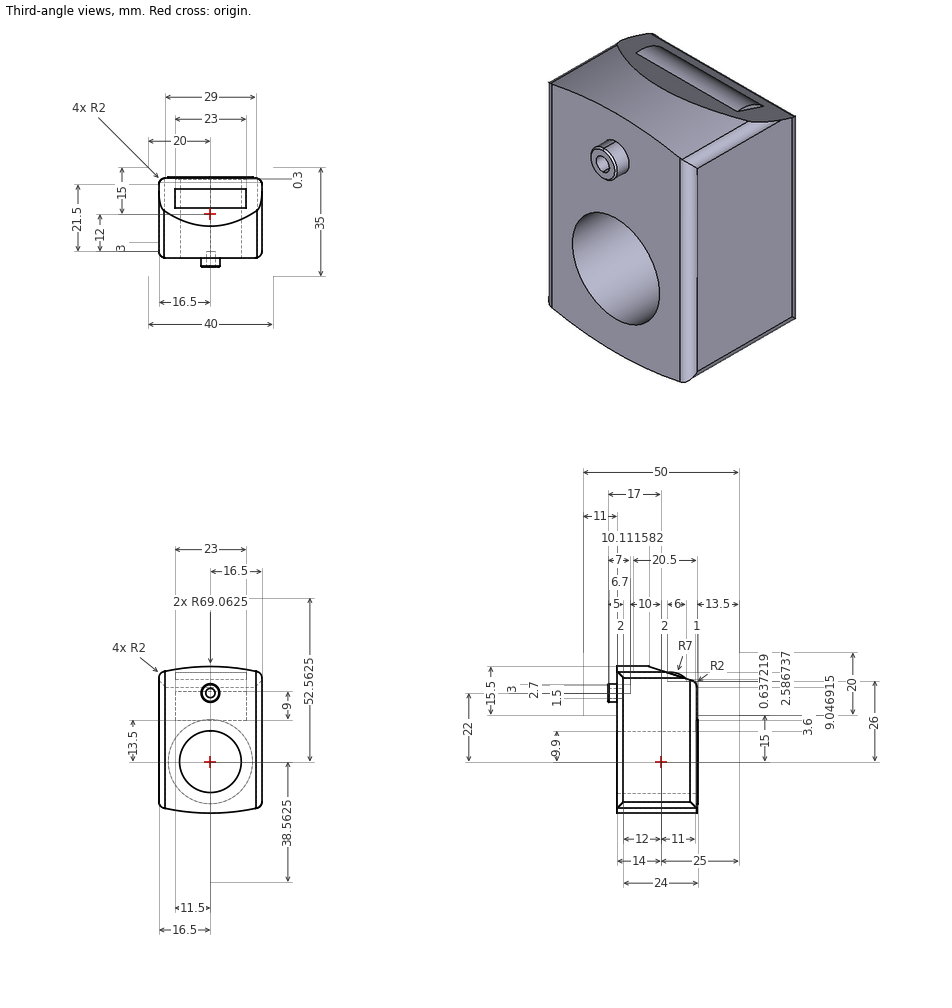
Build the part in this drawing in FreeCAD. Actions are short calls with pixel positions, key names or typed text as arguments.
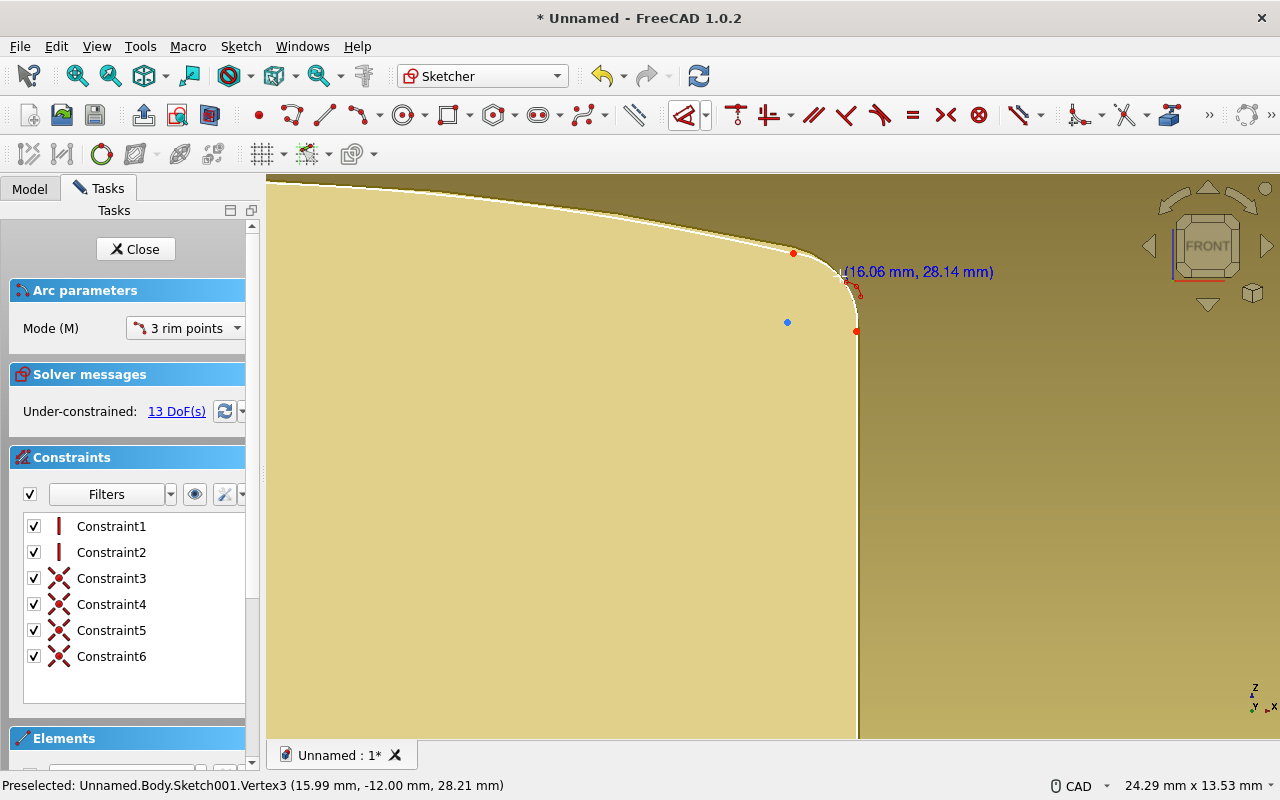
scroll(840, 279, down, 8)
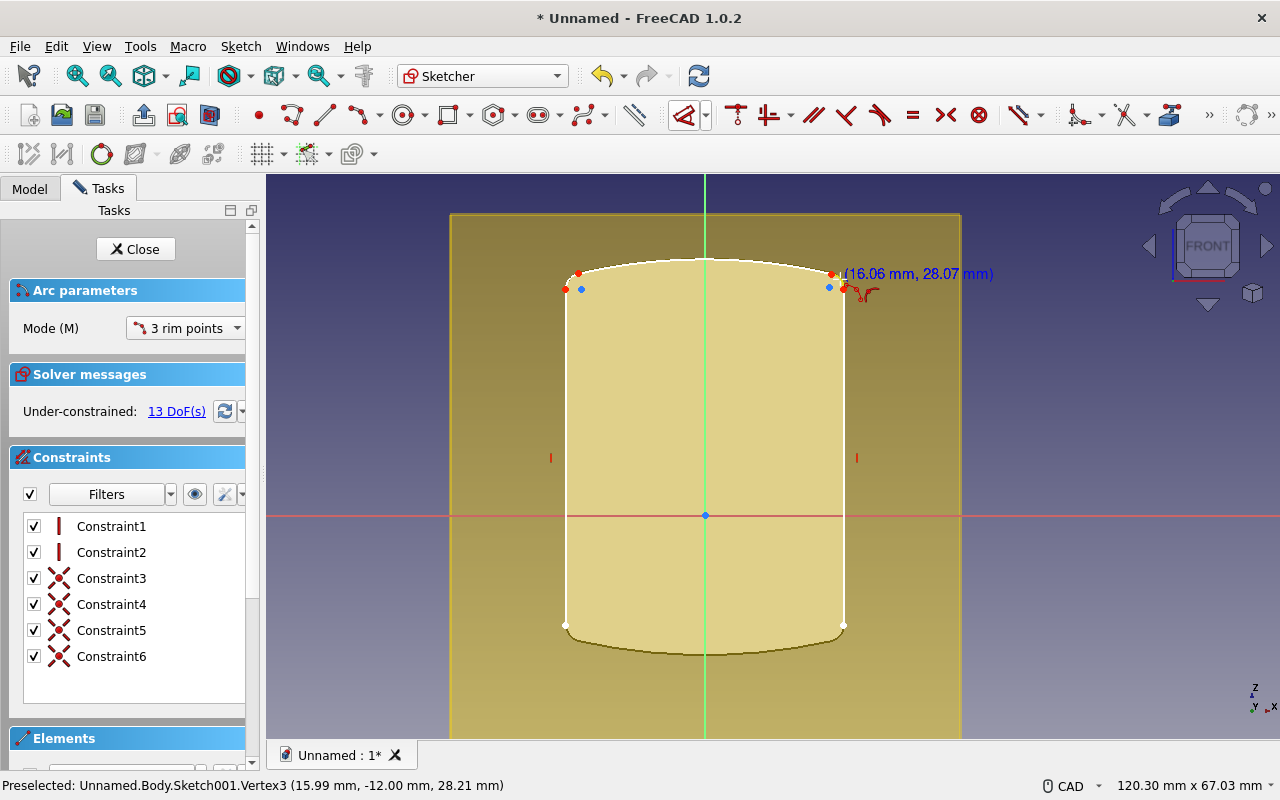
click(844, 626)
click(831, 641)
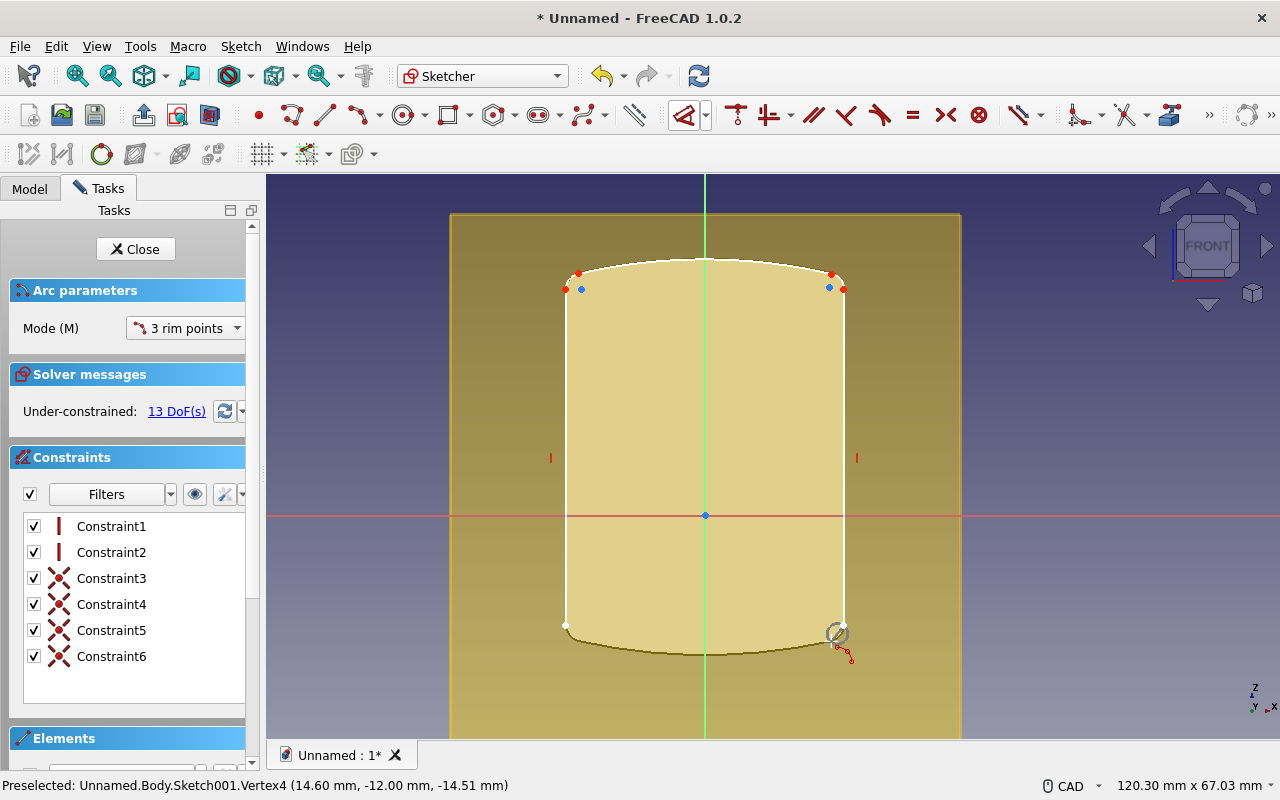
scroll(840, 635, up, 8)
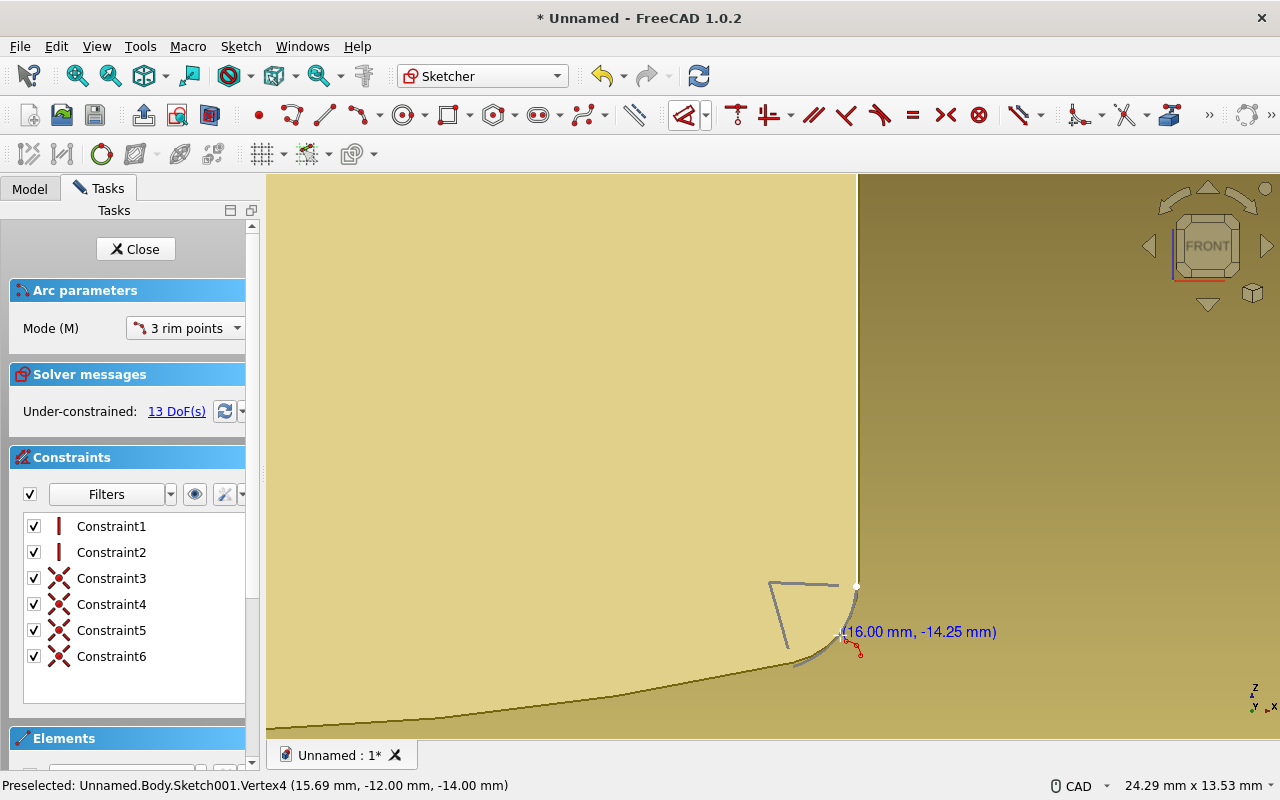
click(840, 633)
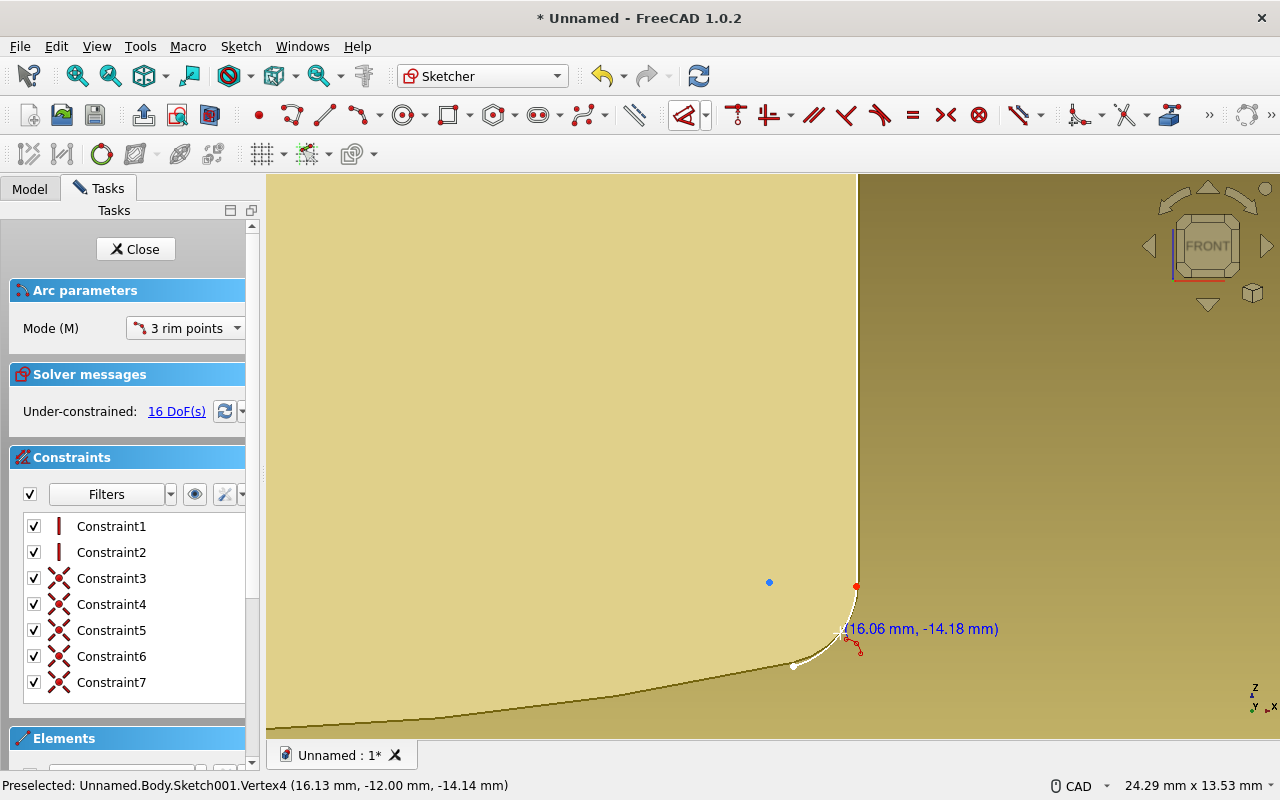
scroll(840, 635, down, 8)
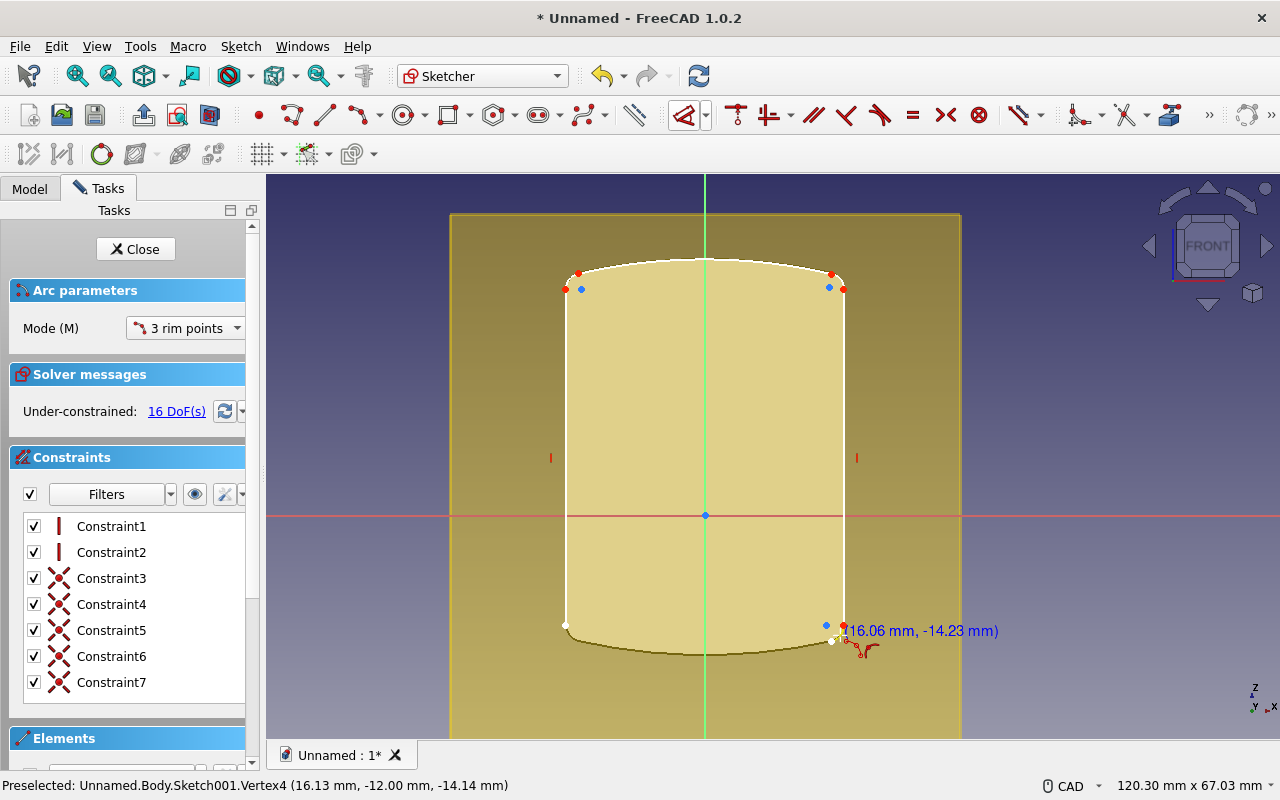
click(831, 642)
click(579, 641)
click(680, 654)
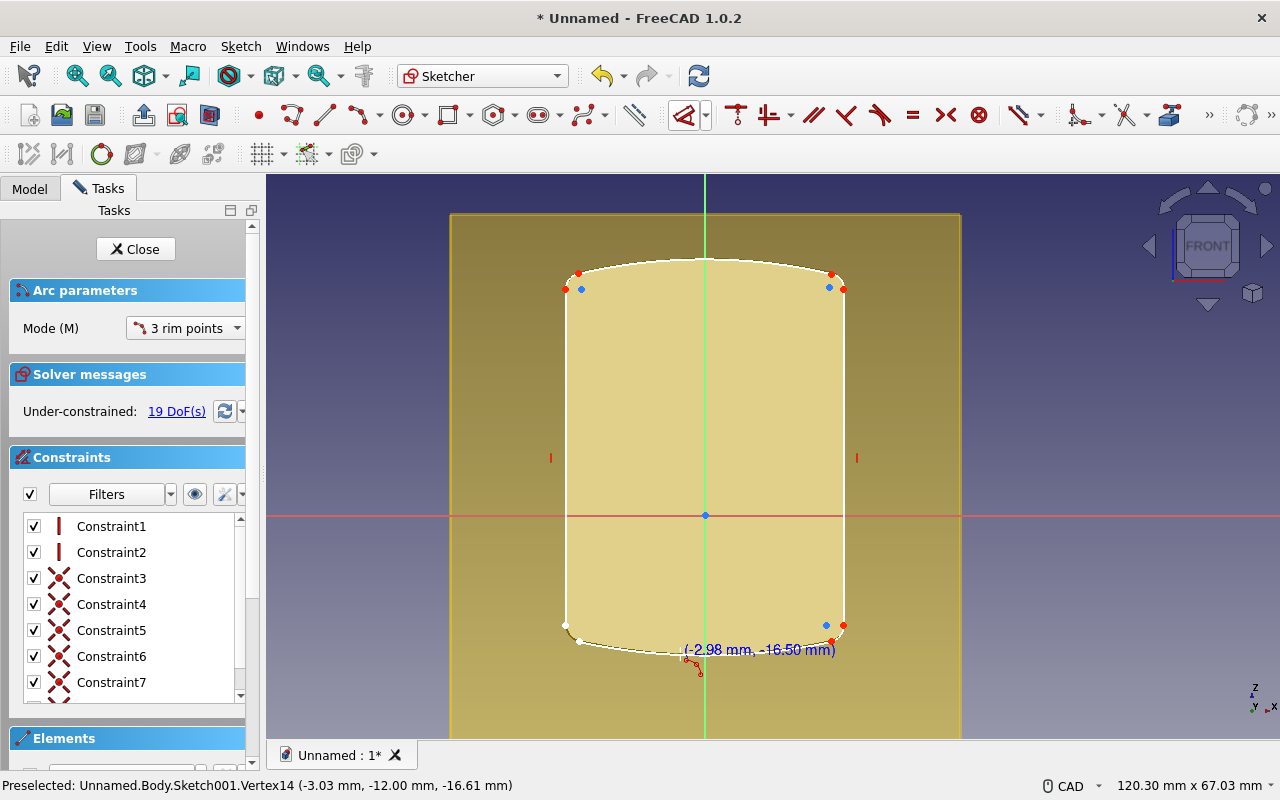
click(579, 642)
click(566, 626)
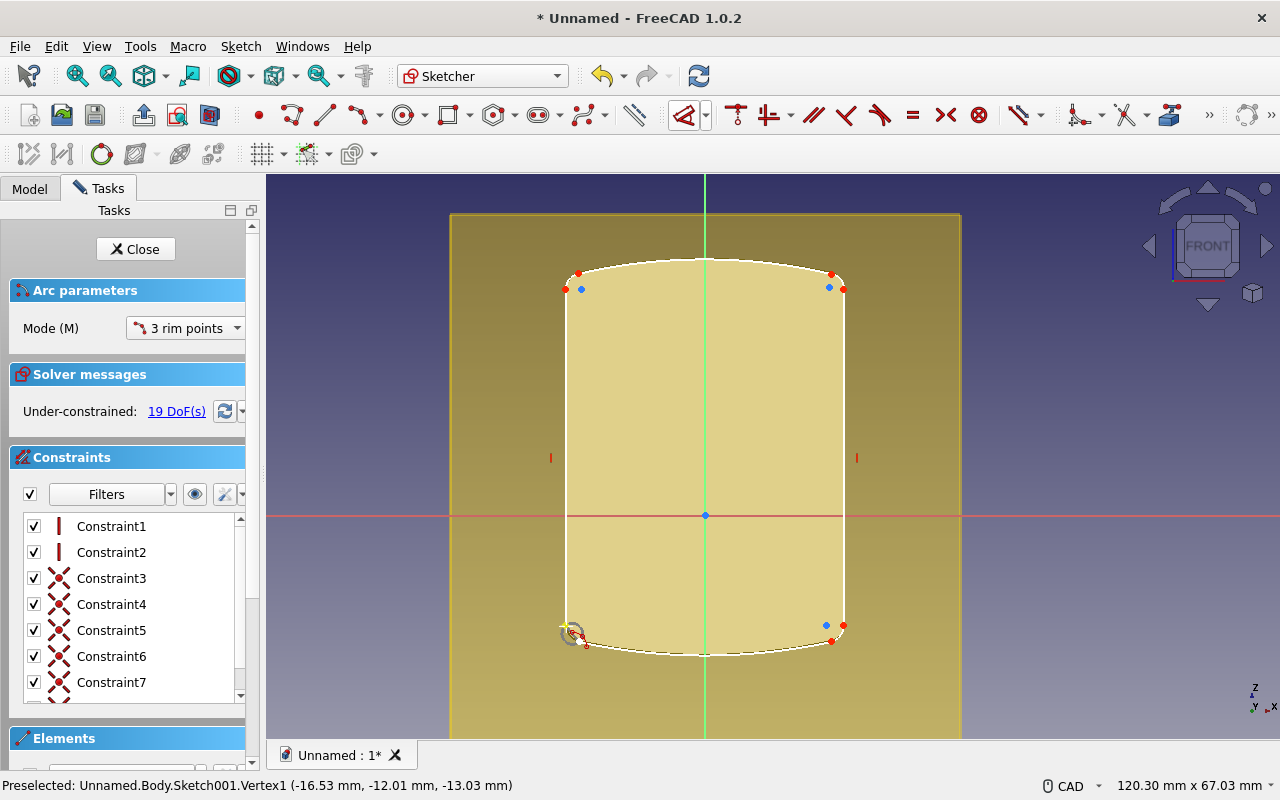
scroll(570, 635, up, 8)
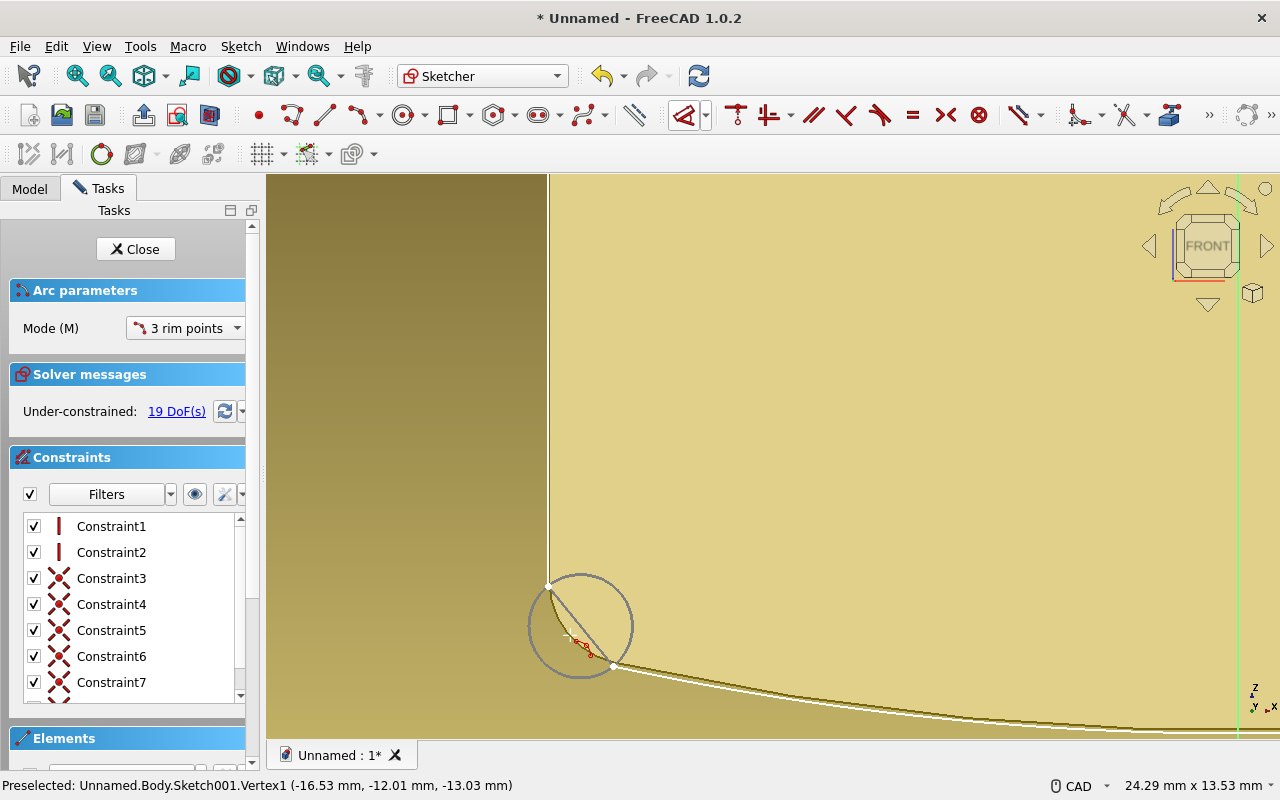
click(568, 633)
key(Escape)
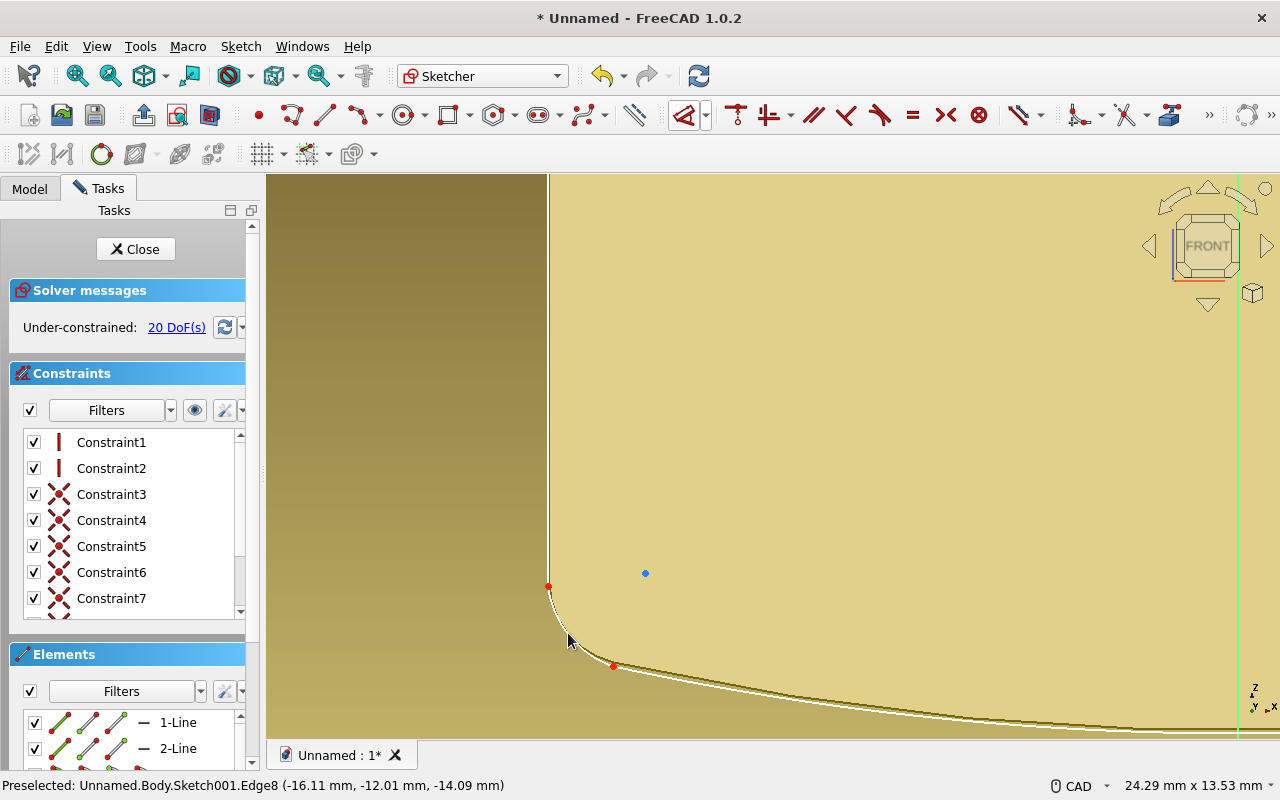
scroll(570, 635, down, 8)